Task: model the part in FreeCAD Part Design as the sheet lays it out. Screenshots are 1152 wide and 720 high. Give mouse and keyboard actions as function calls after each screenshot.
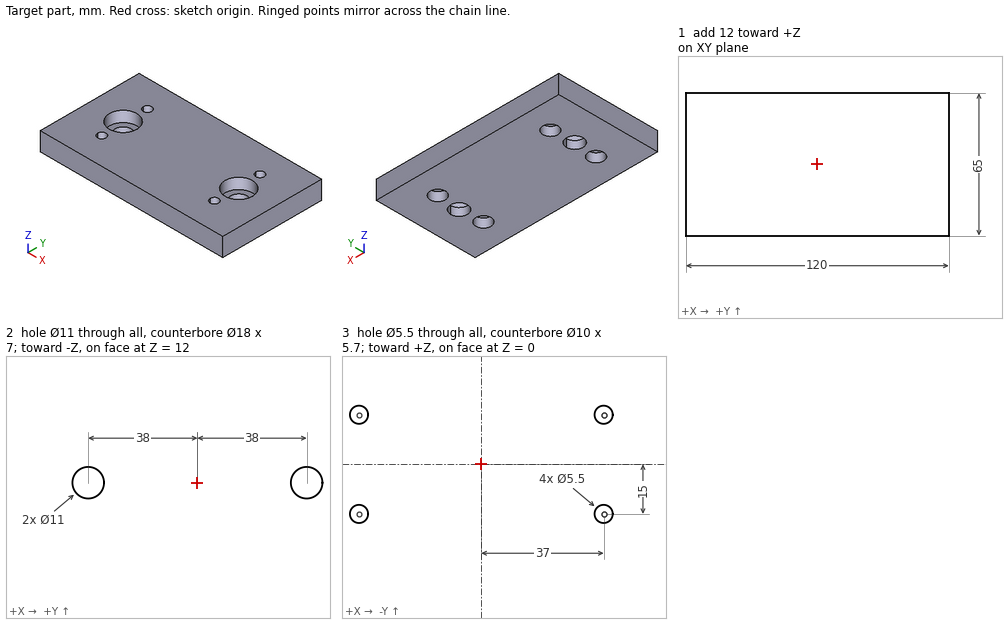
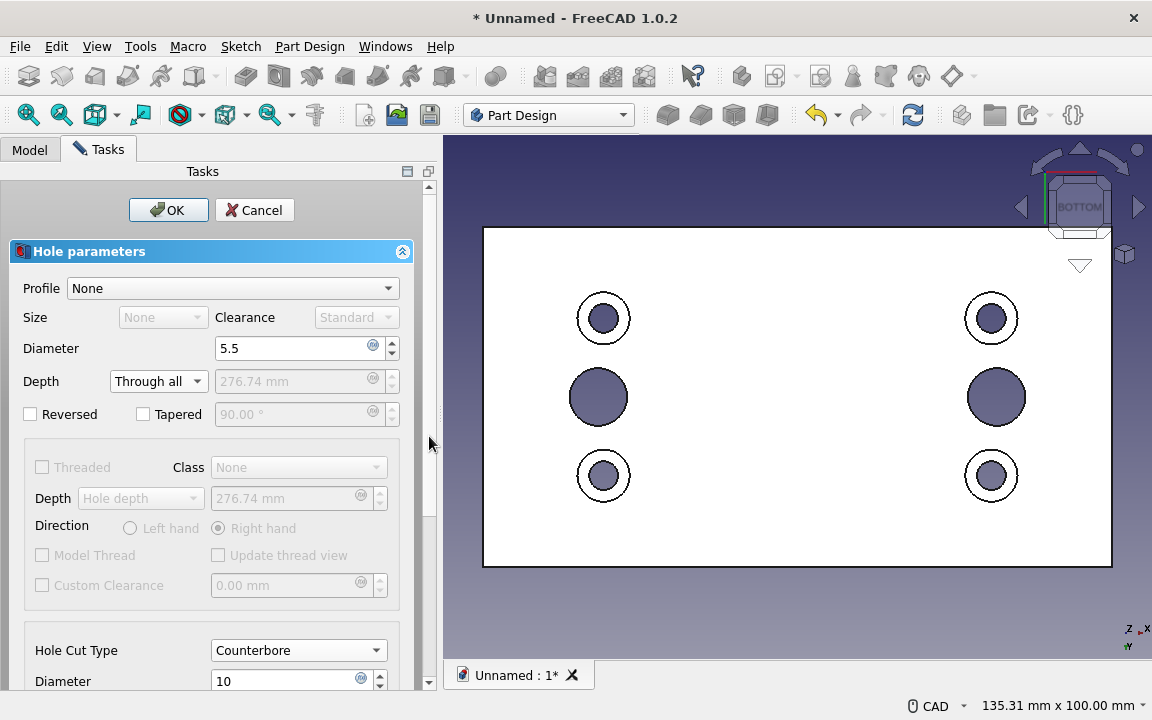
click(169, 210)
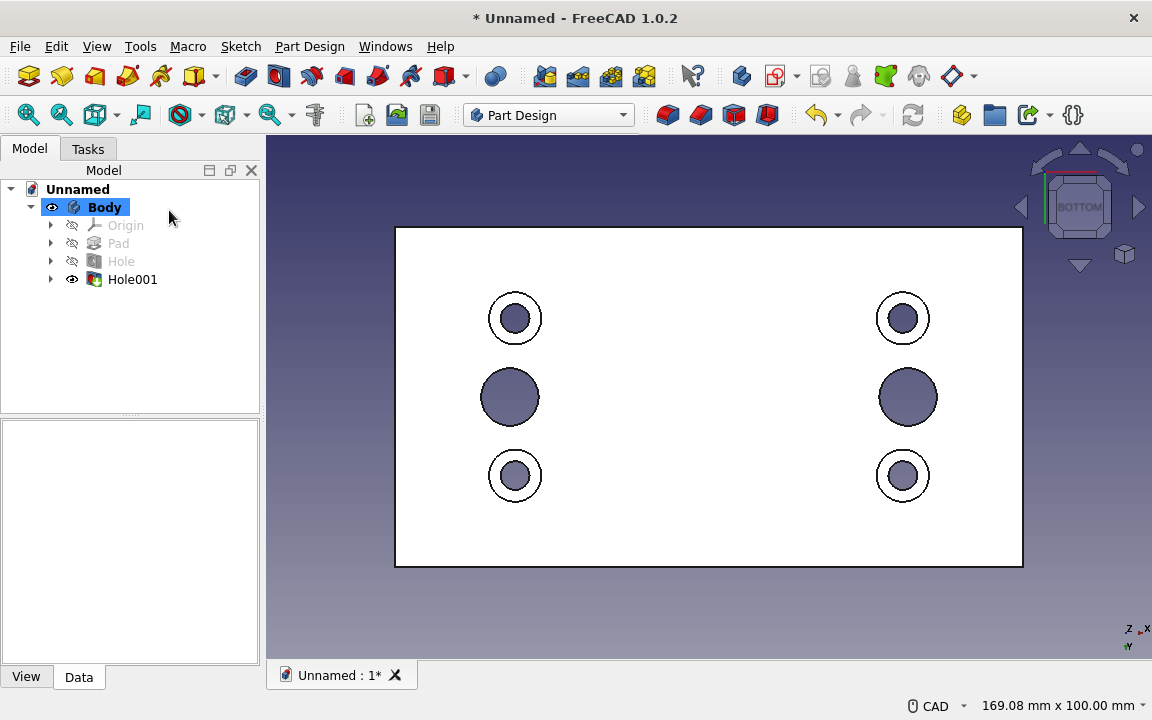
key(0)